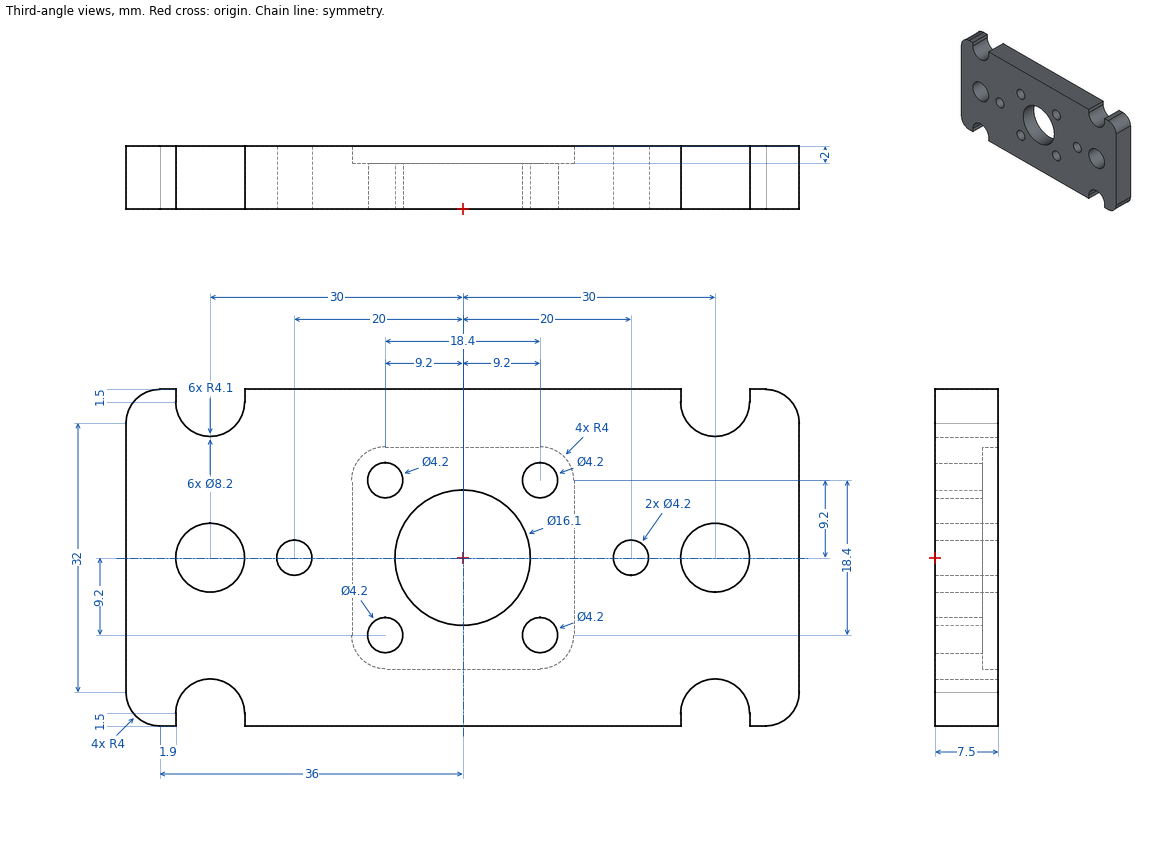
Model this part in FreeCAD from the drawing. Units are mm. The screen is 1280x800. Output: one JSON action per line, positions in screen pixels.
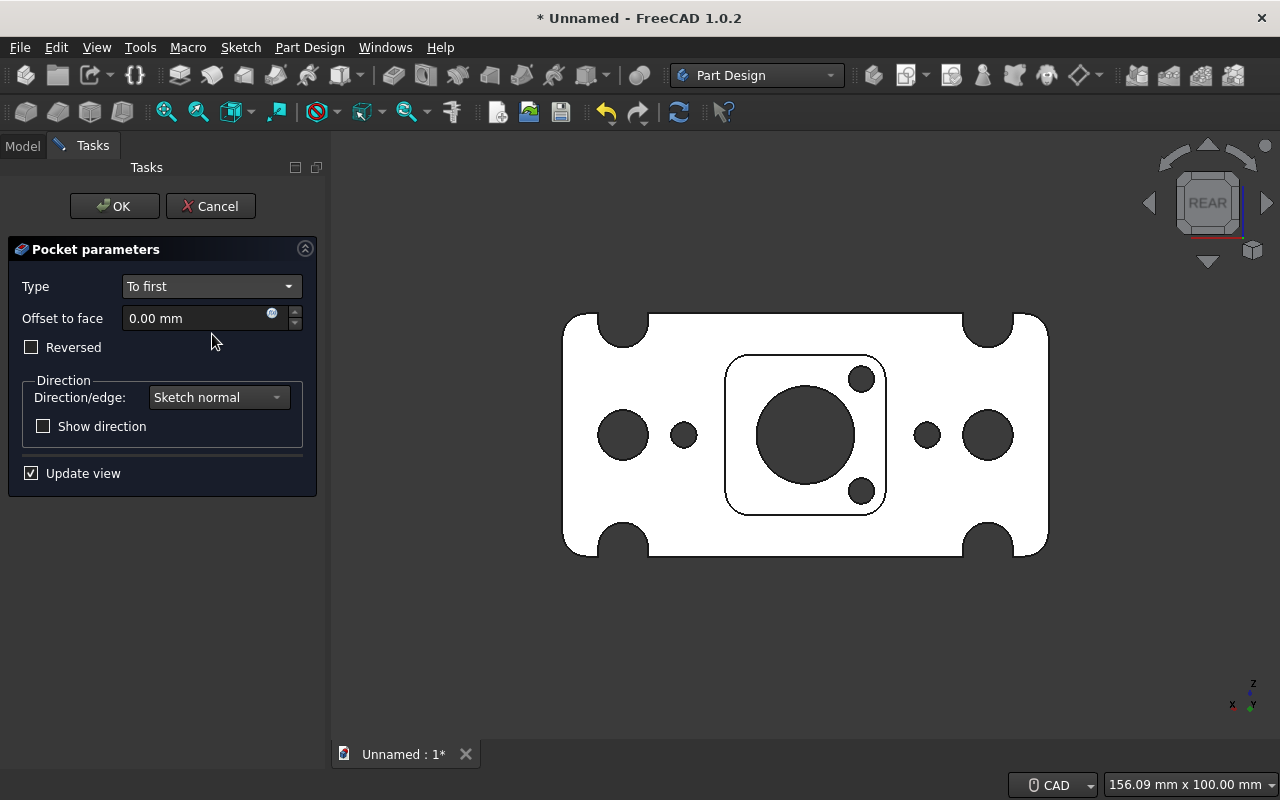
{"action": "left_click", "coordinate": [115, 206]}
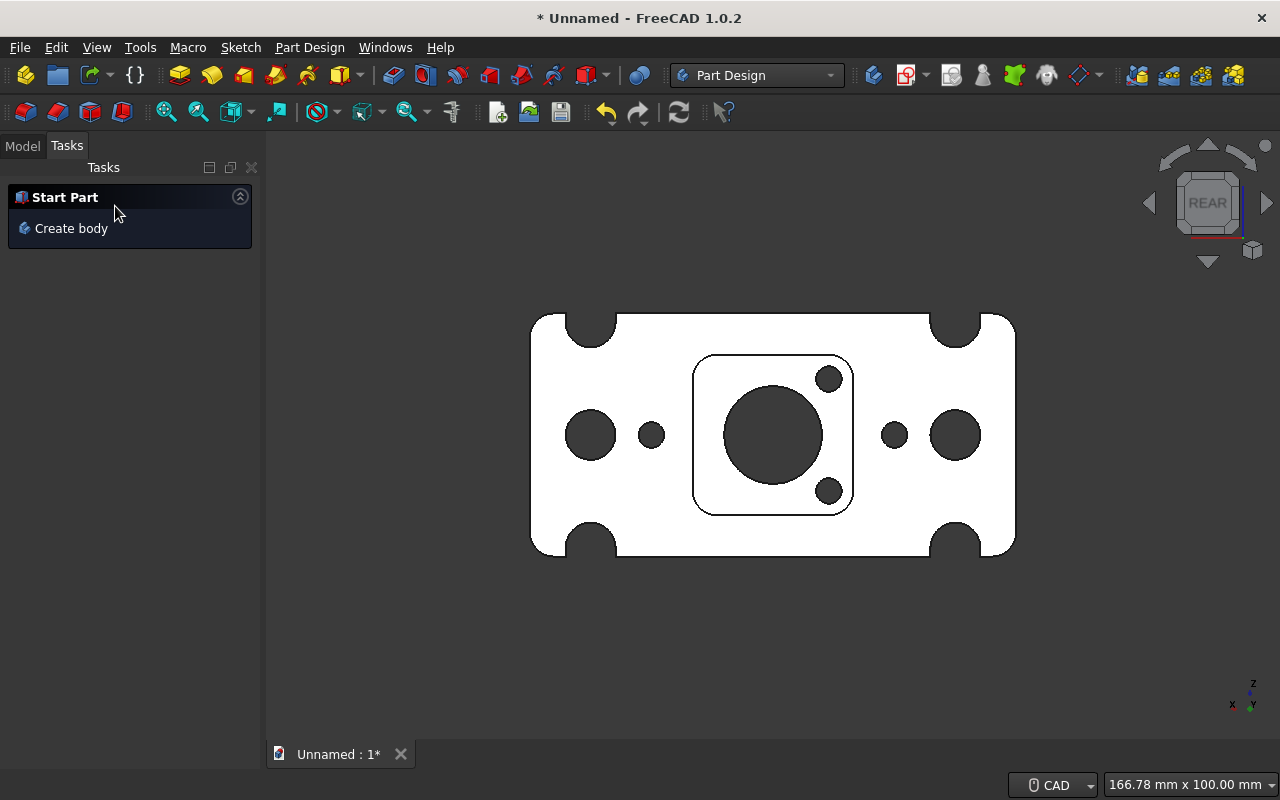
{"action": "left_click", "coordinate": [727, 388]}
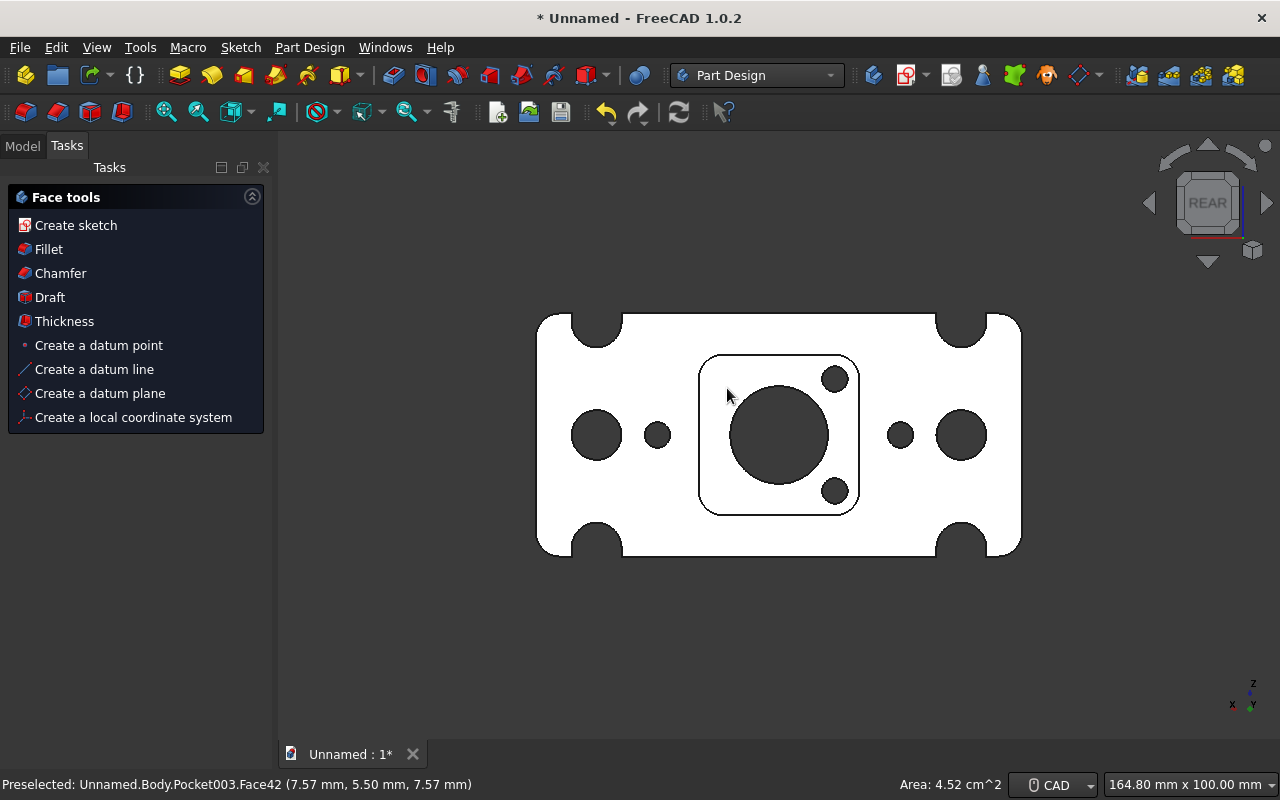
{"action": "left_click", "coordinate": [906, 76]}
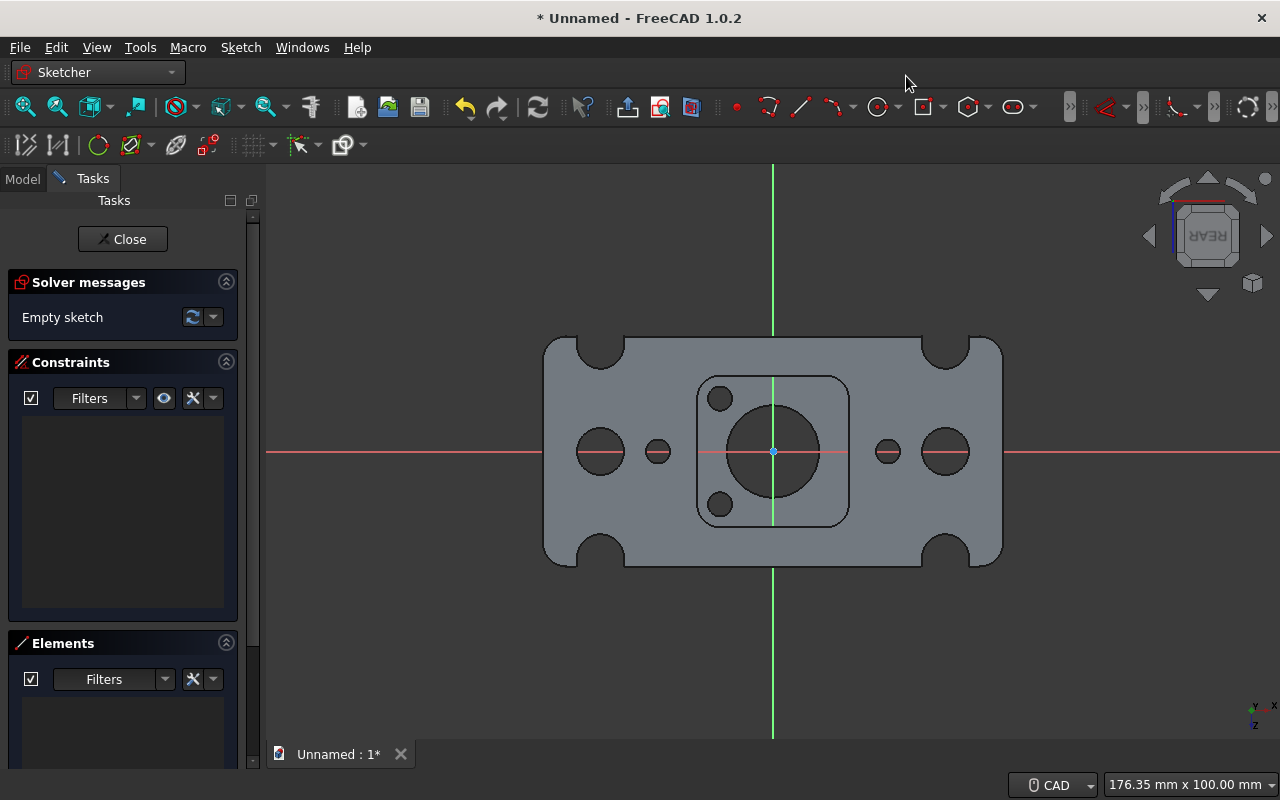
{"action": "scroll", "coordinate": [834, 508], "scroll_direction": "up", "scroll_amount": 14}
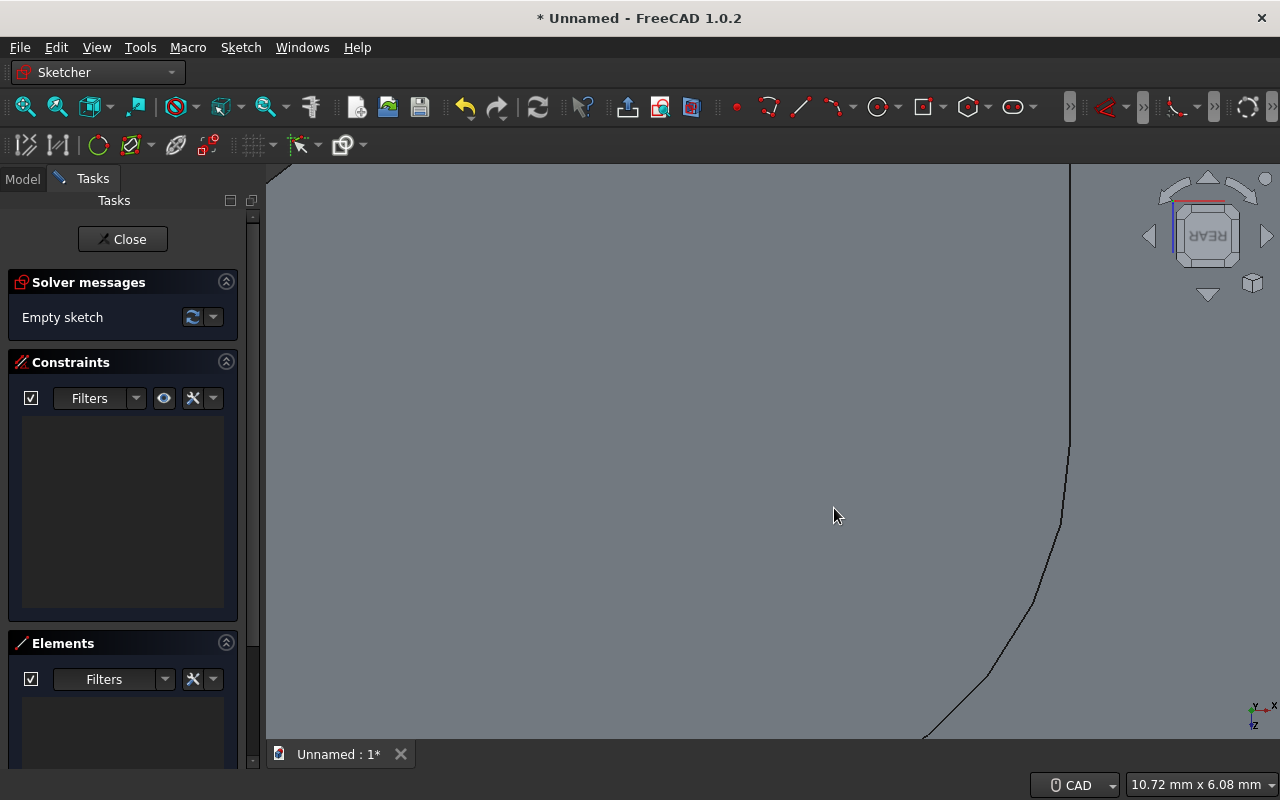
{"action": "left_click", "coordinate": [878, 108]}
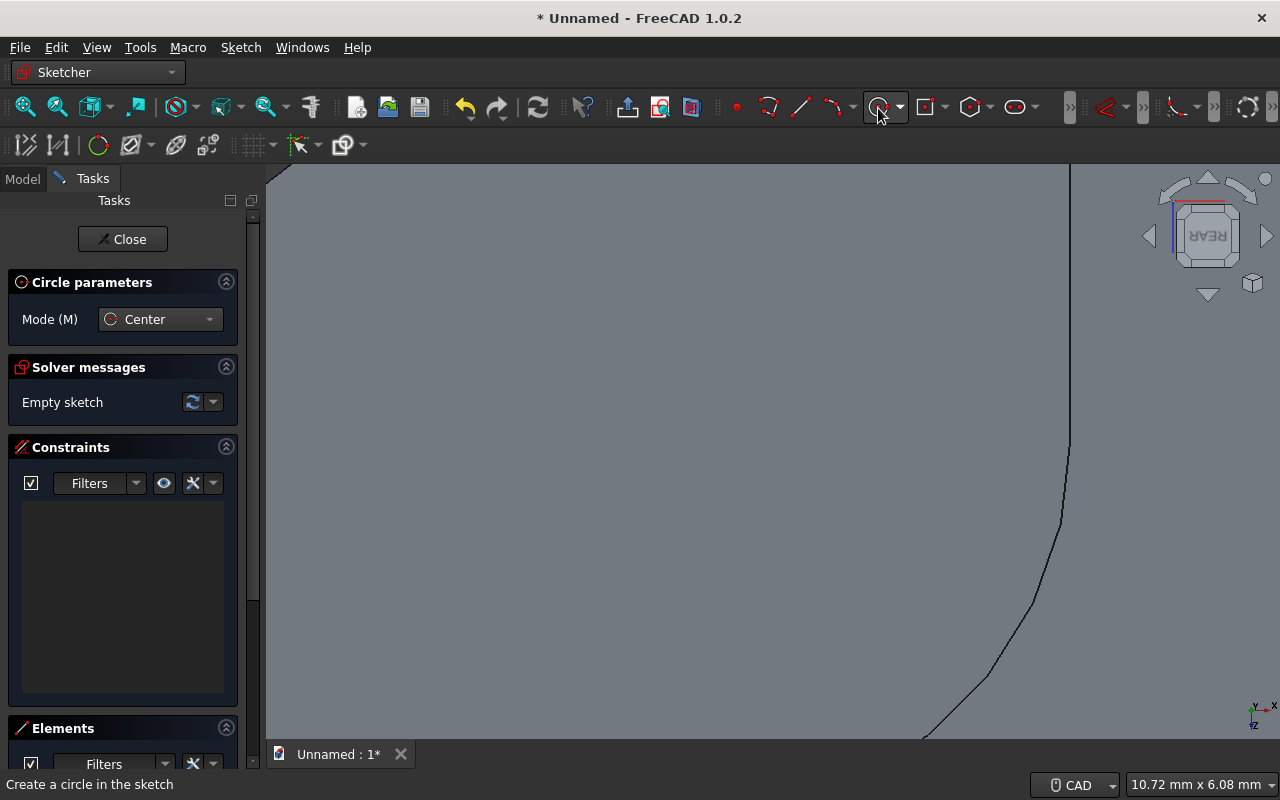
{"action": "left_click", "coordinate": [692, 440]}
{"action": "mouse_move", "coordinate": [833, 299]}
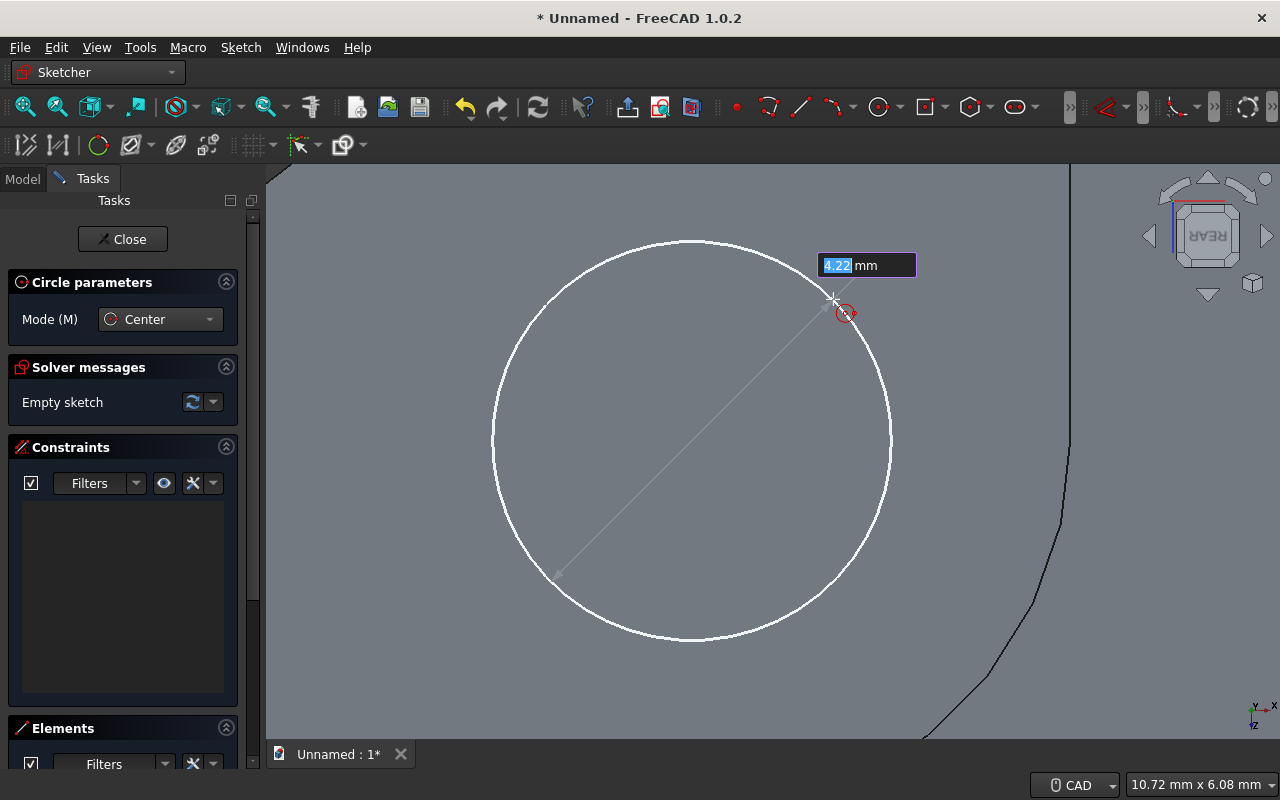
{"action": "type", "text": "4.2"}
{"action": "key", "text": "Return"}
{"action": "key", "text": "Escape"}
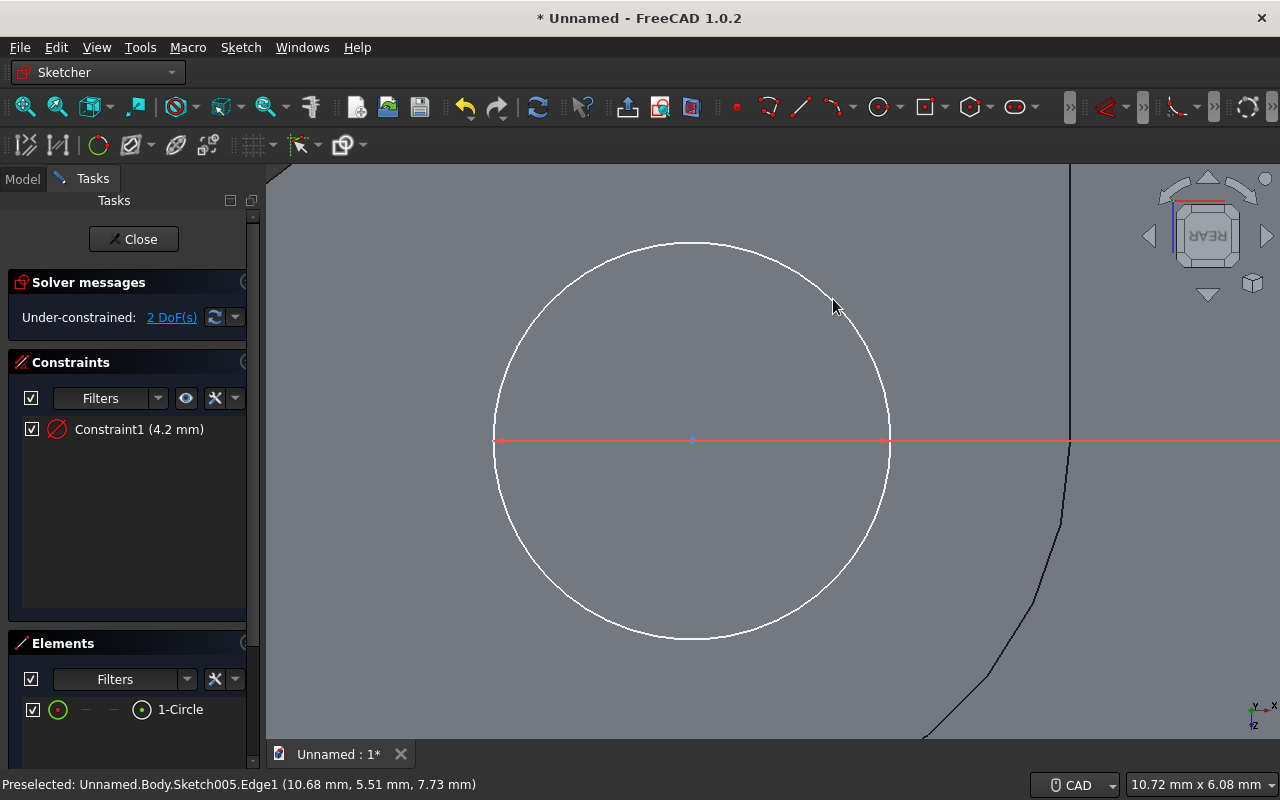
{"action": "left_click", "coordinate": [1106, 108]}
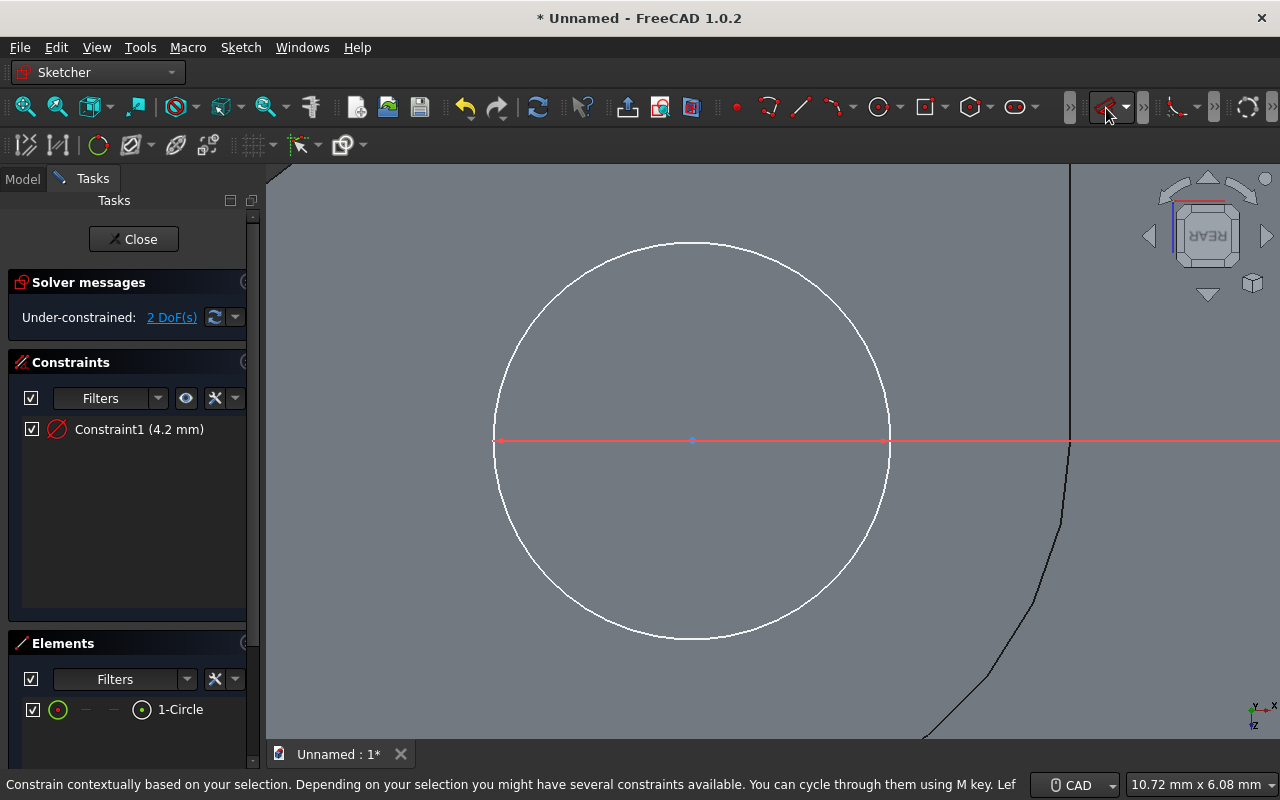
{"action": "left_click", "coordinate": [692, 441]}
{"action": "left_click", "coordinate": [401, 475]}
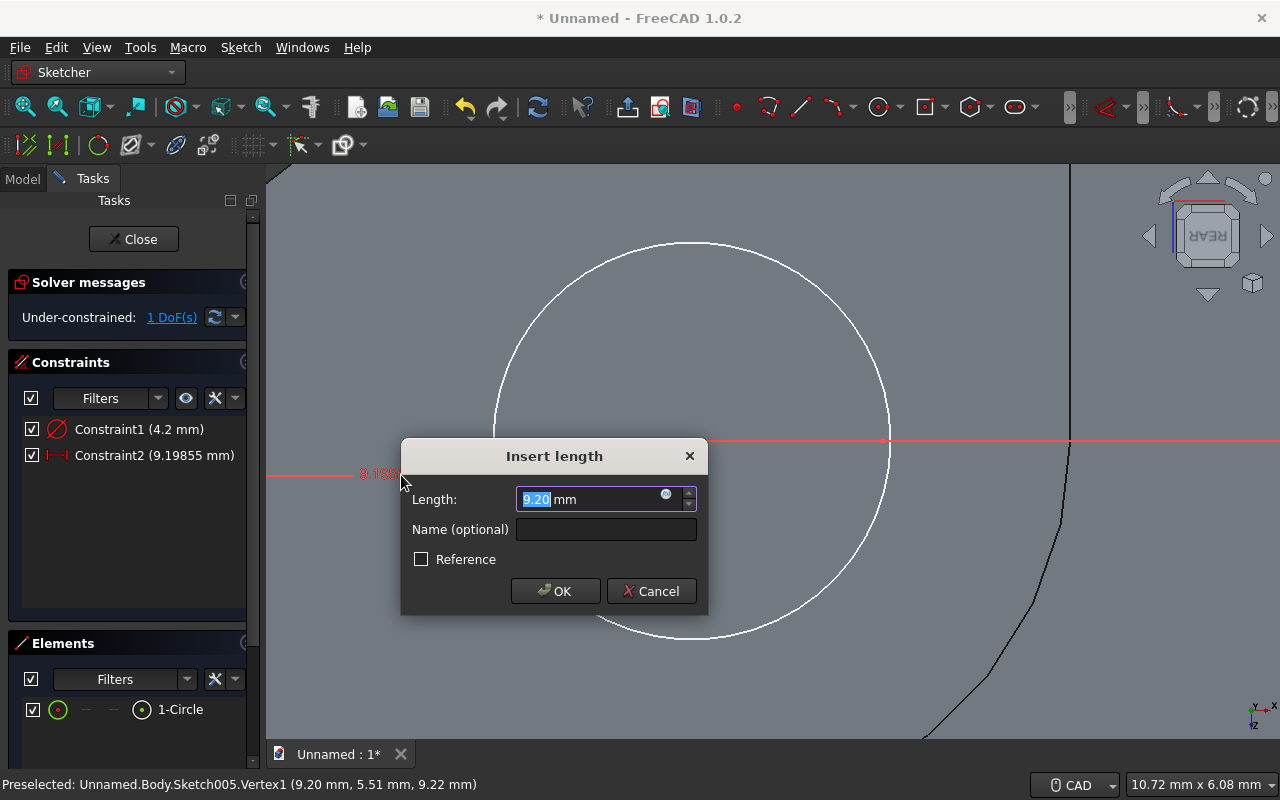
{"action": "type", "text": "9.2"}
{"action": "key", "text": "Return"}